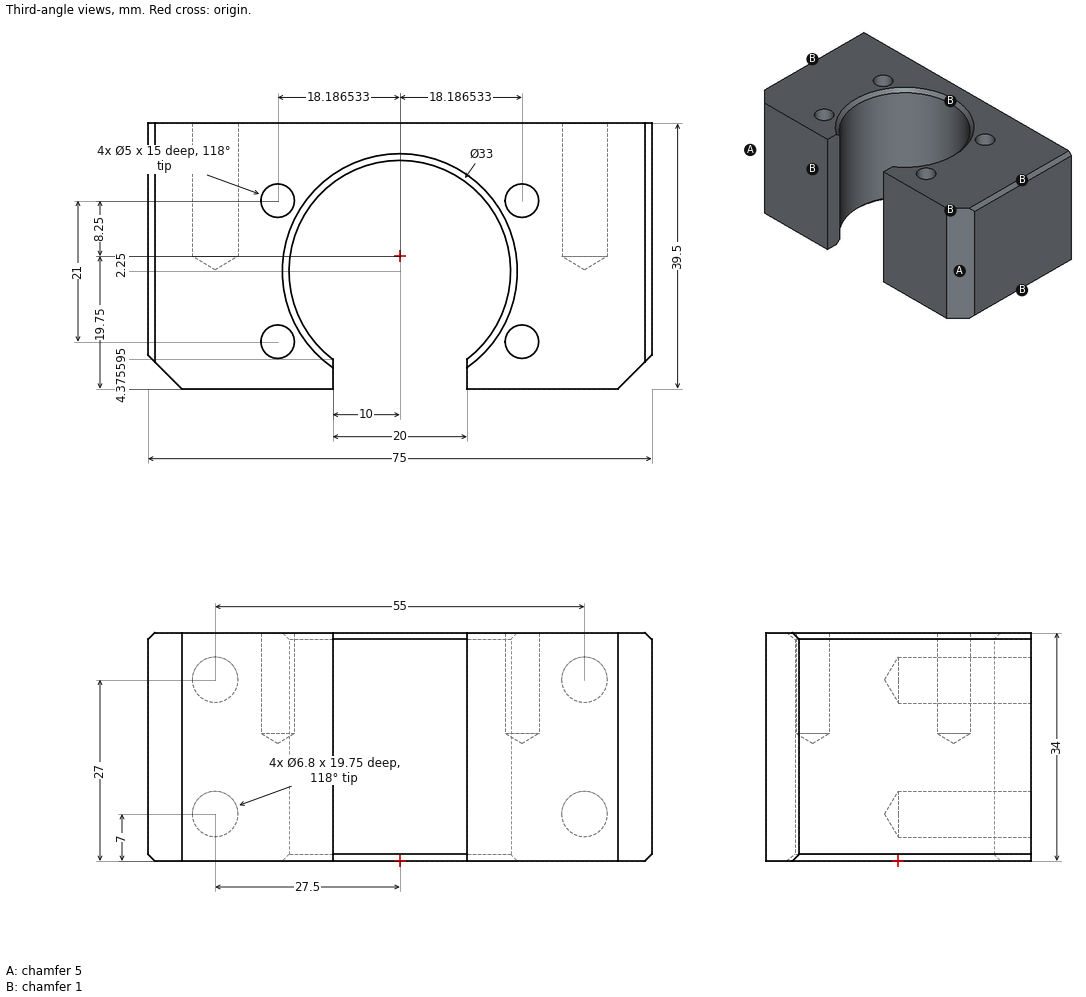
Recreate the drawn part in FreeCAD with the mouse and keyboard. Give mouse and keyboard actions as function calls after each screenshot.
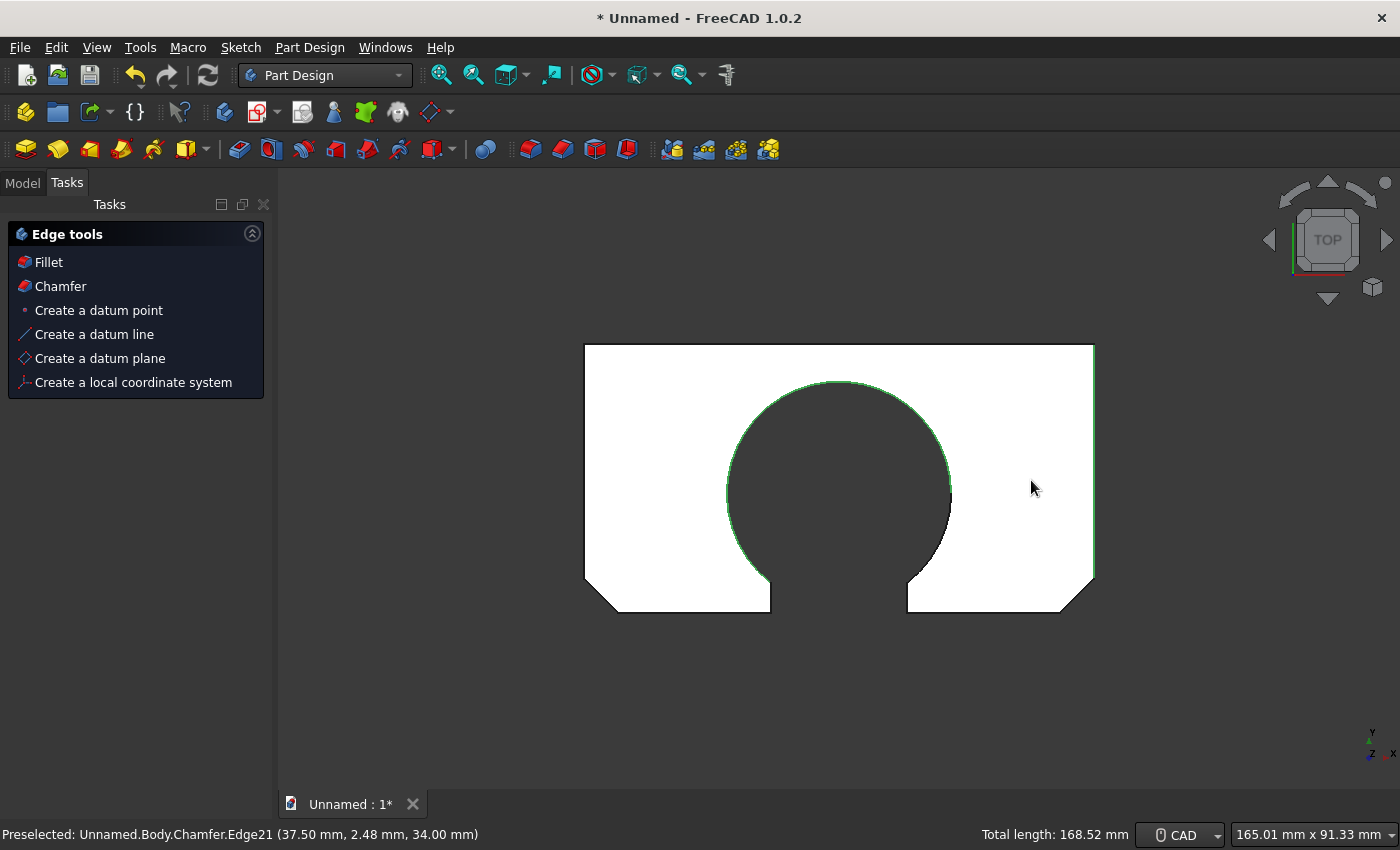
click(584, 461, ctrl)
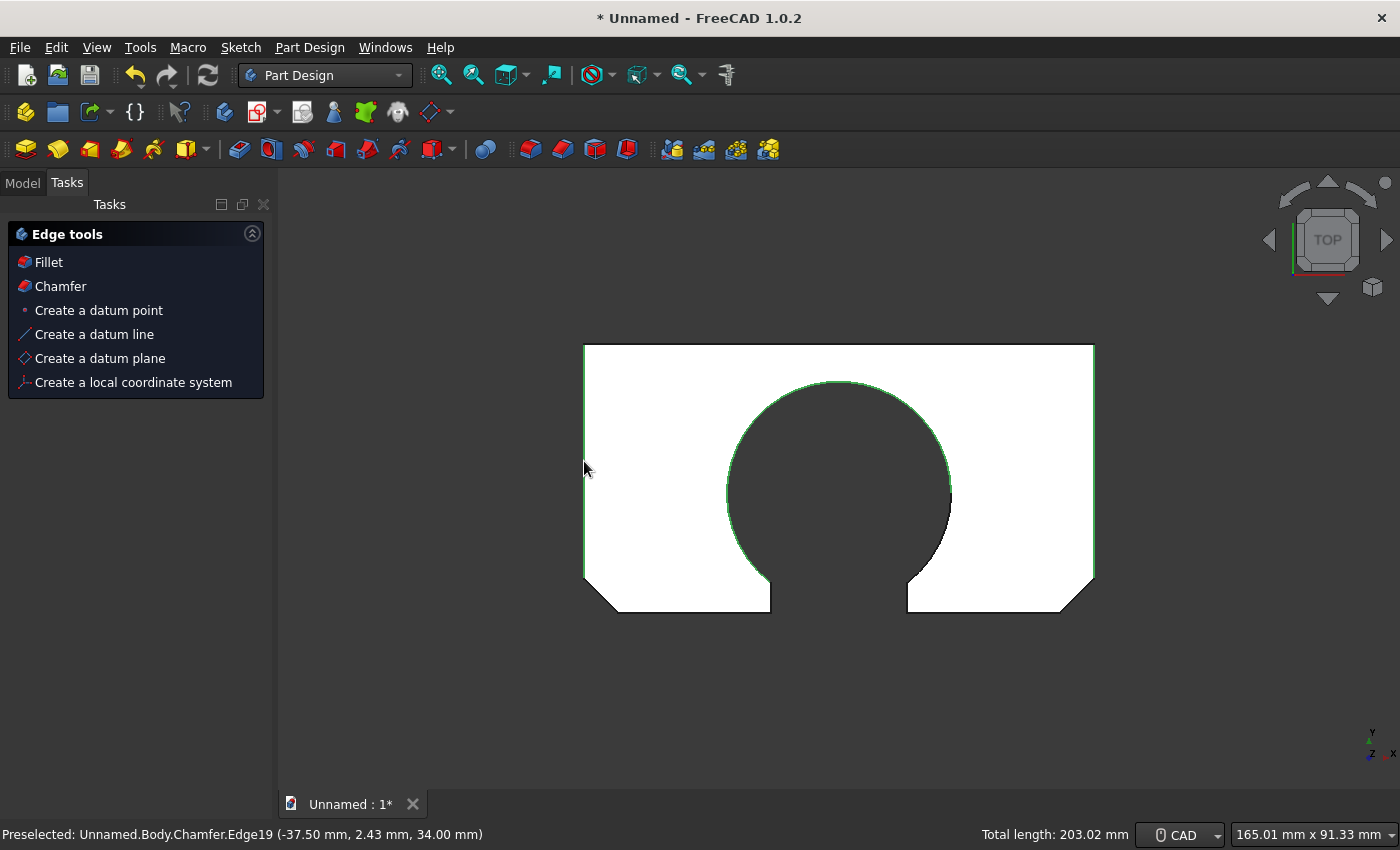
key(1)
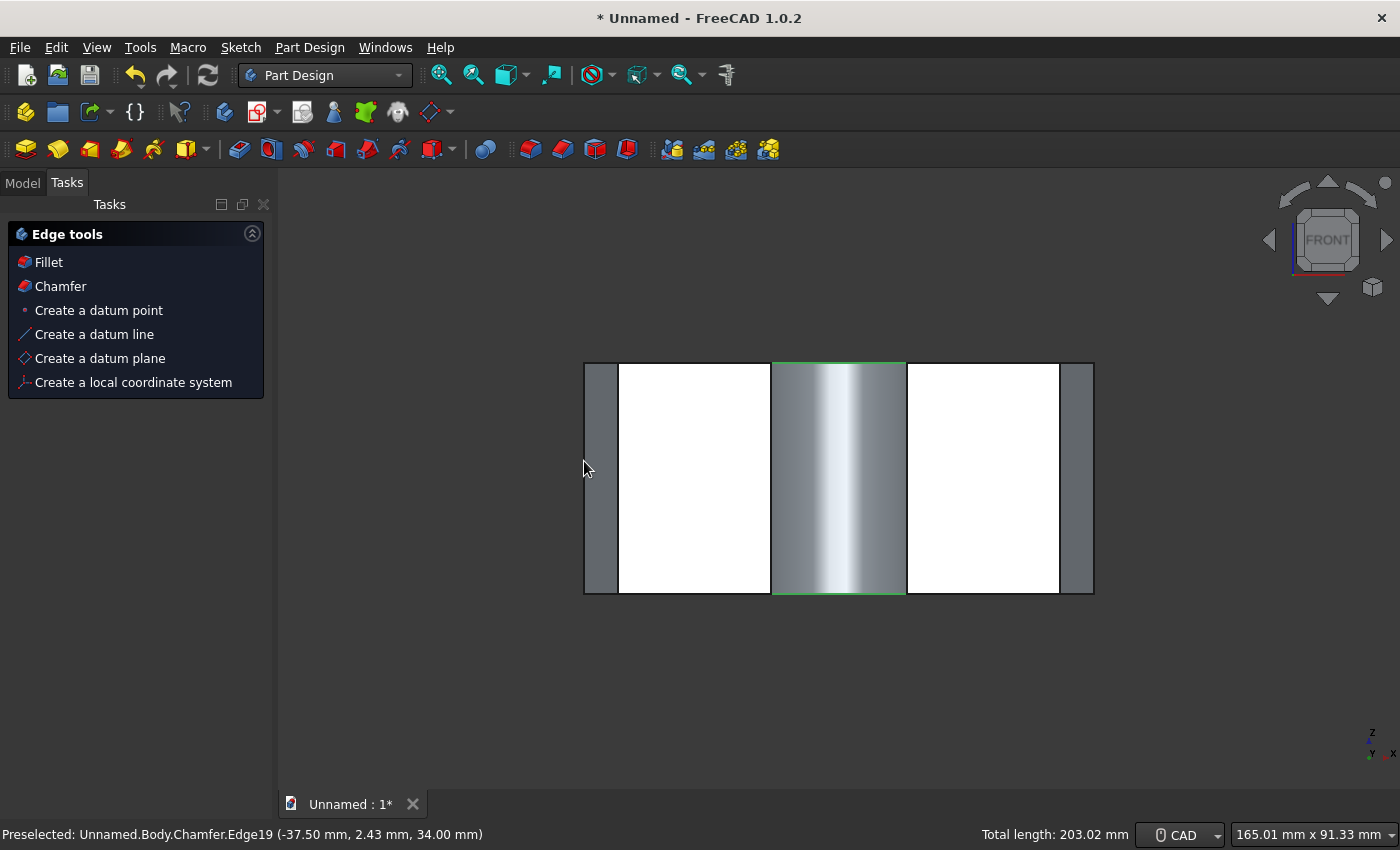
key(3)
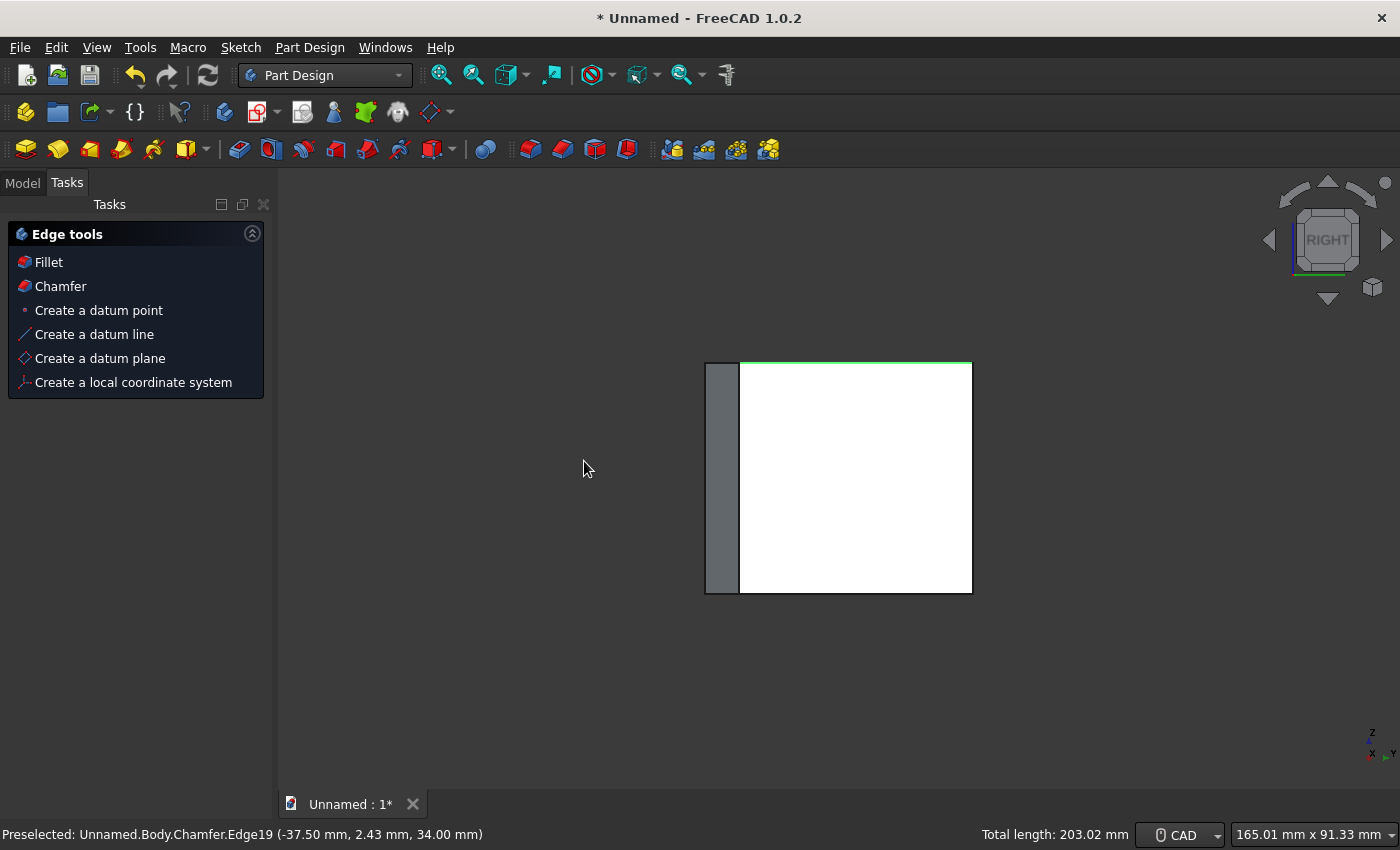
key(v)
key(f)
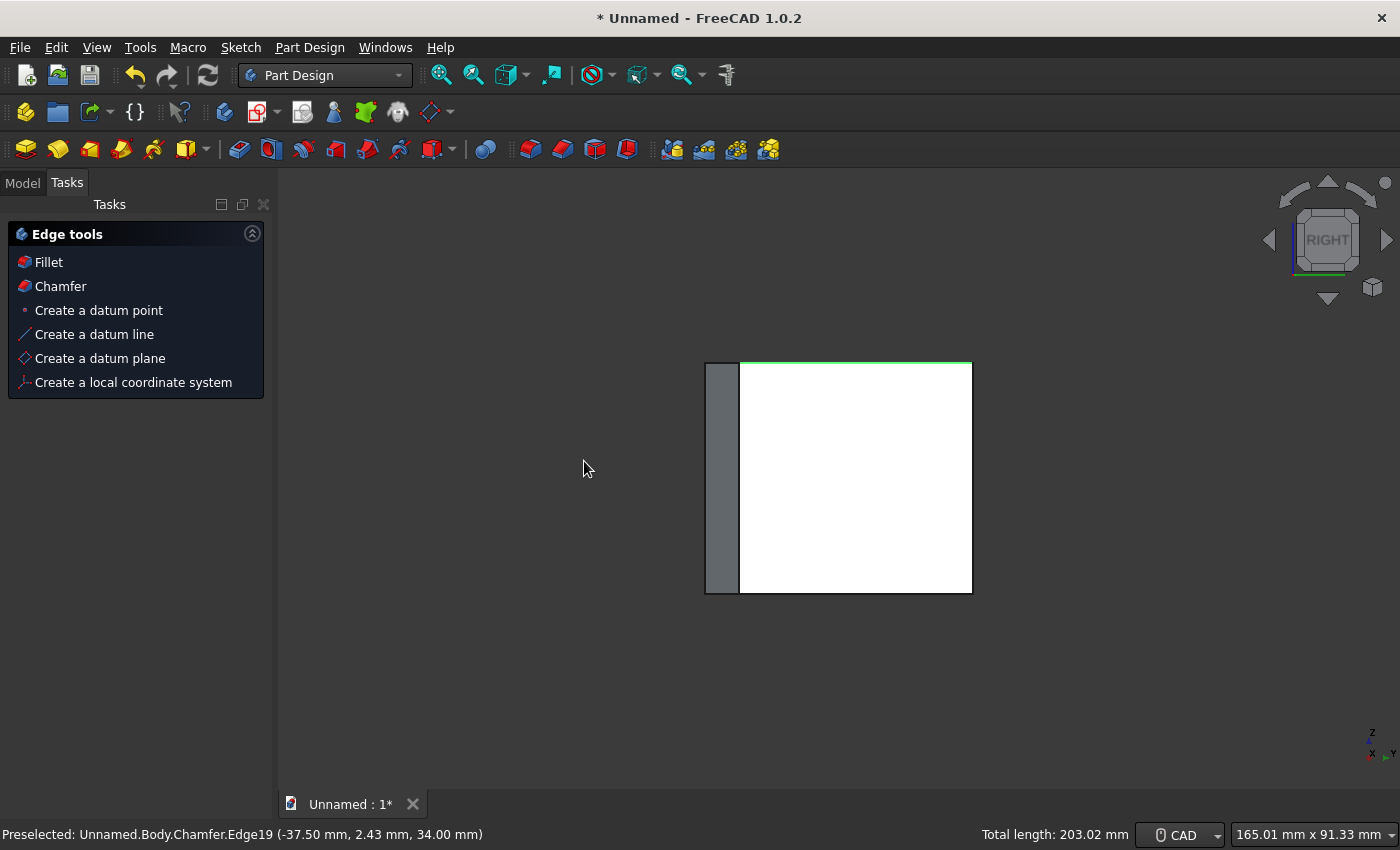
click(856, 593, ctrl)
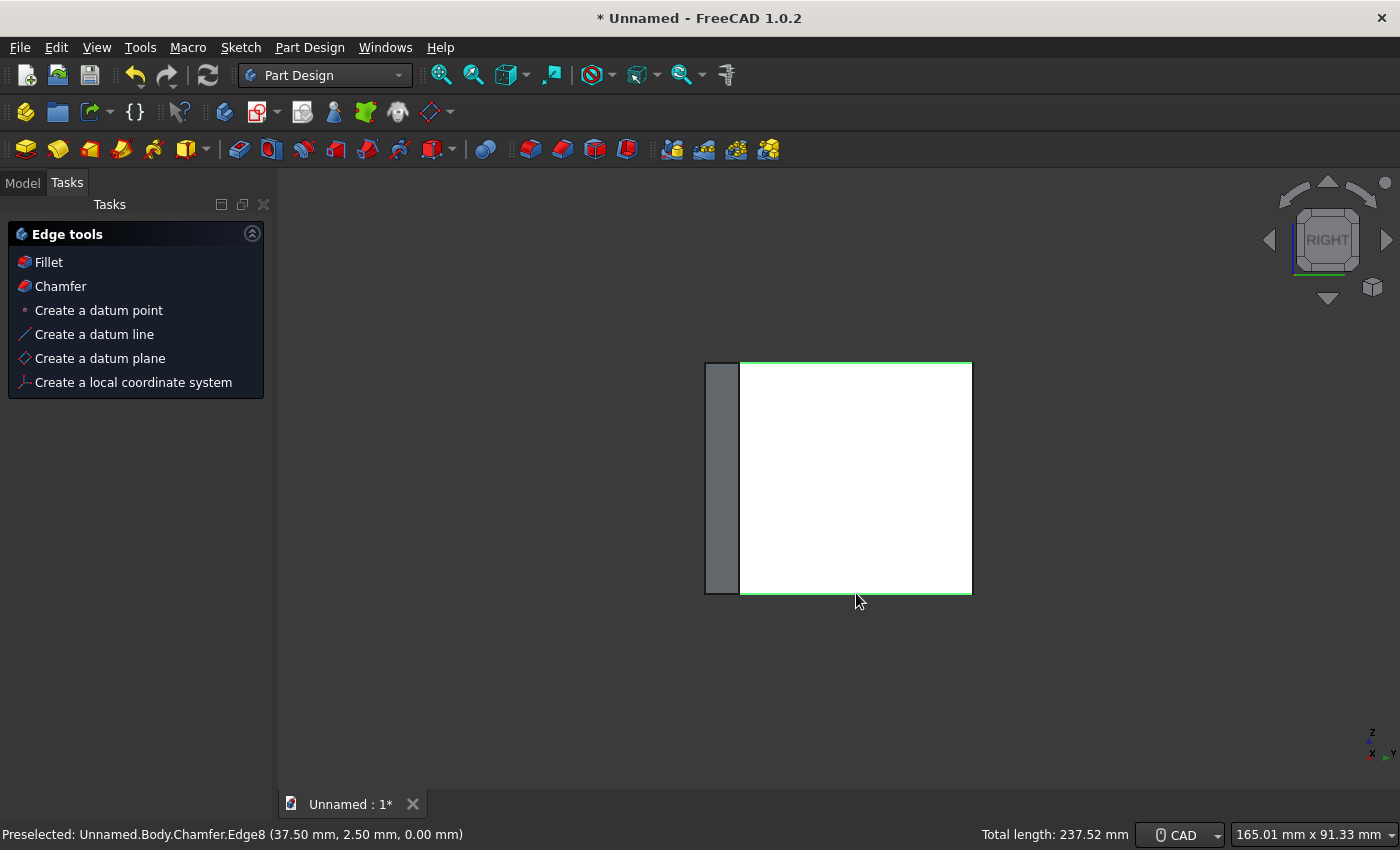
key(5)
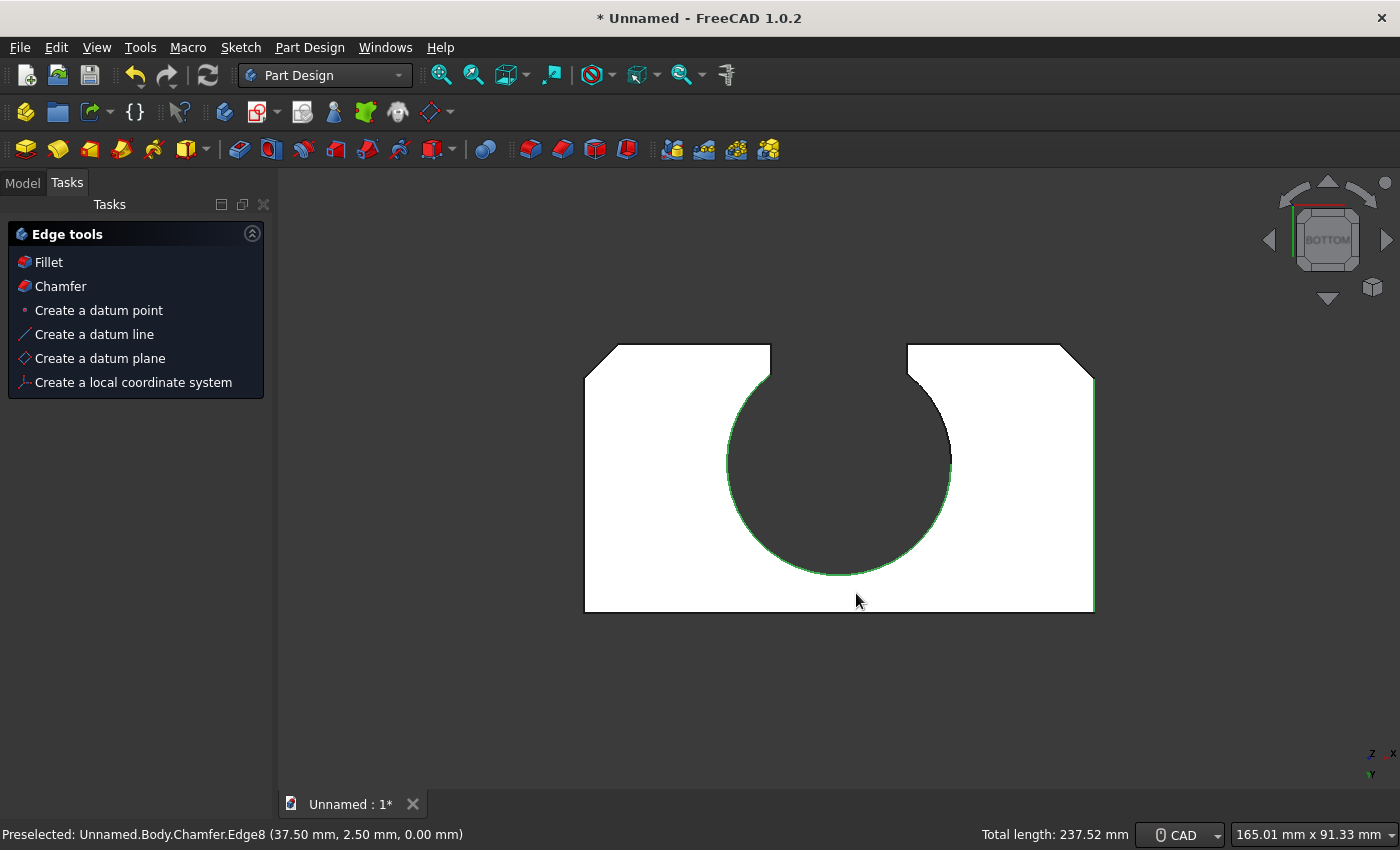
key(4)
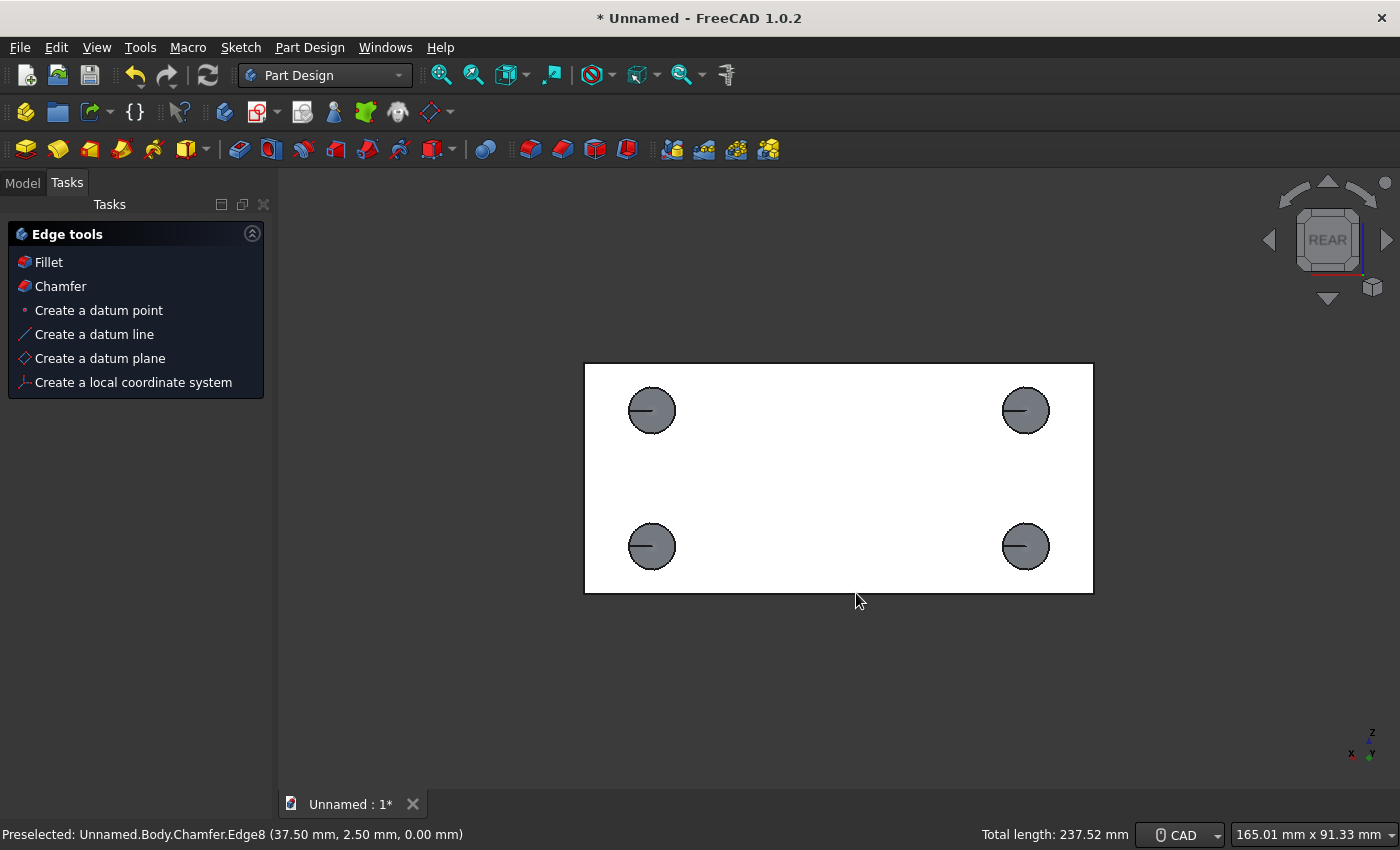
key(6)